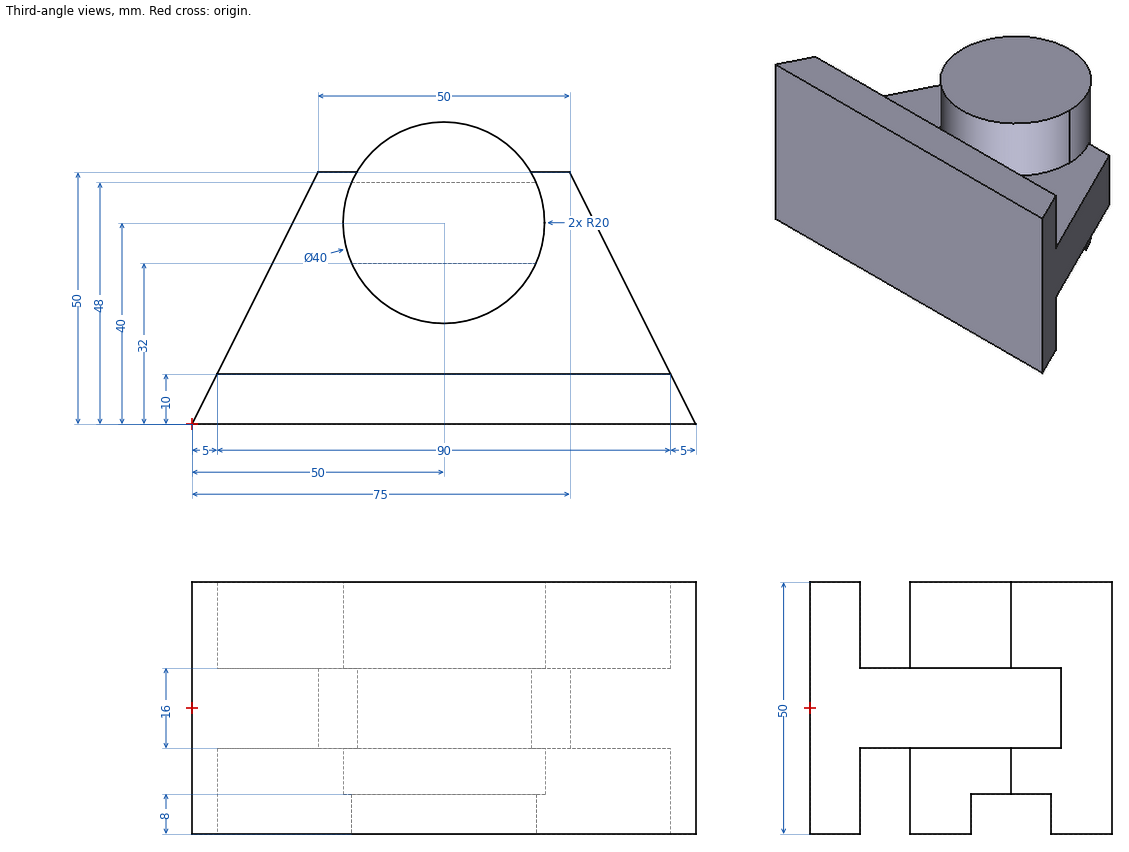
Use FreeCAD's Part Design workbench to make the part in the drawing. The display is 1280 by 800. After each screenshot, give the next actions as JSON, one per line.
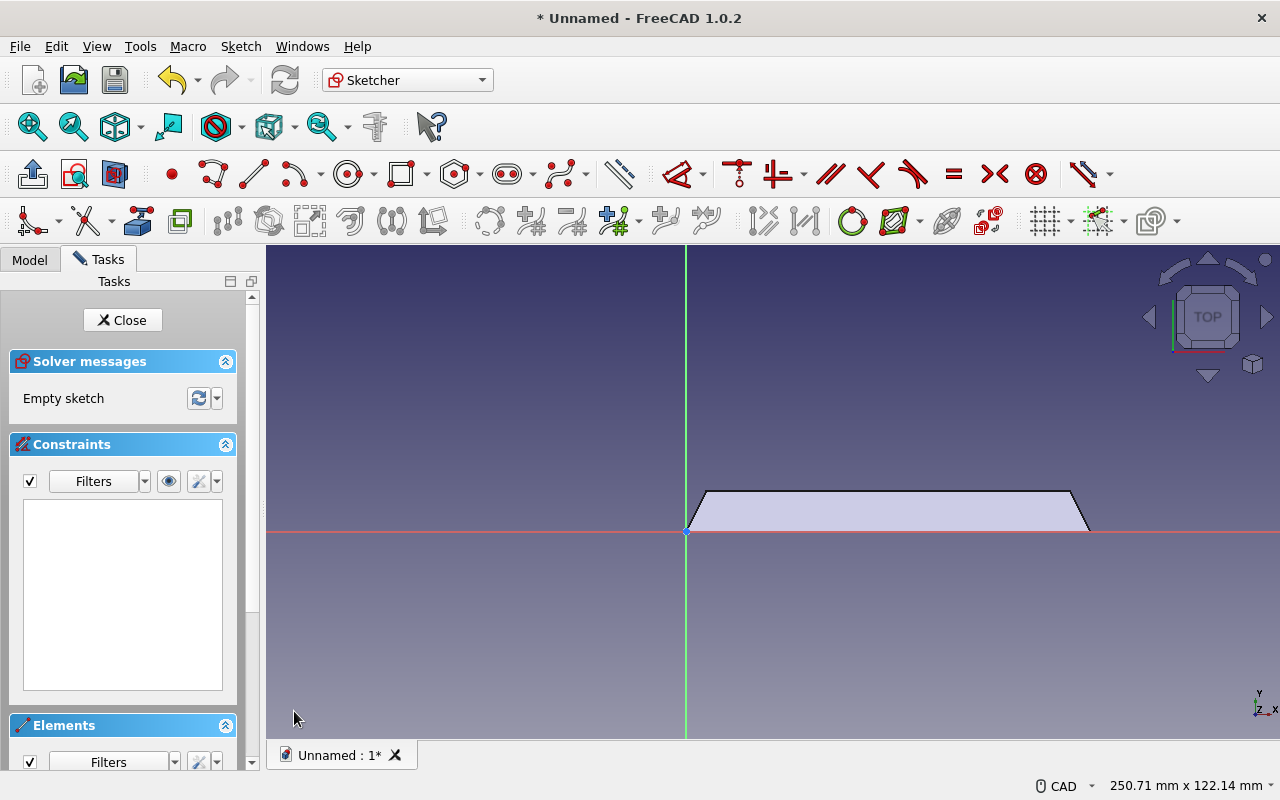
{"action": "scroll", "coordinate": [1115, 306], "scroll_direction": "up", "scroll_amount": 2}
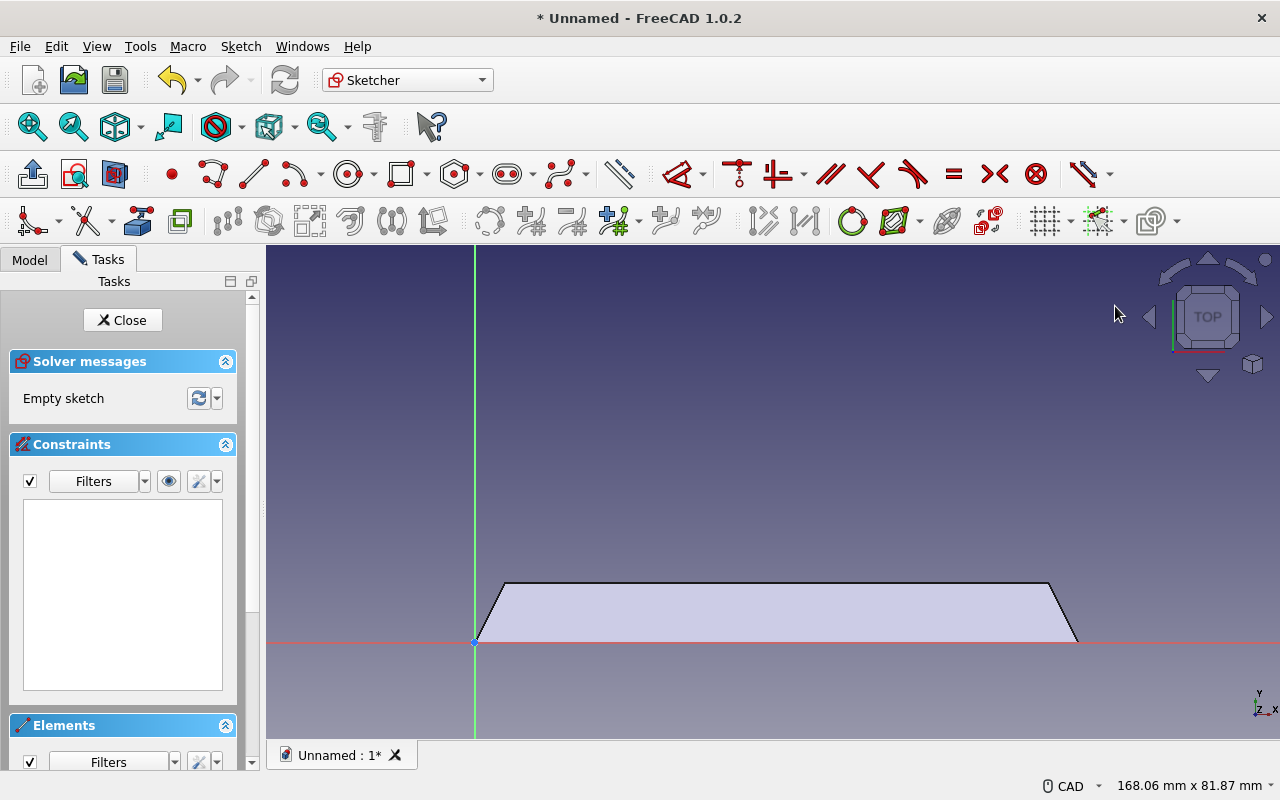
{"action": "left_click", "coordinate": [213, 174]}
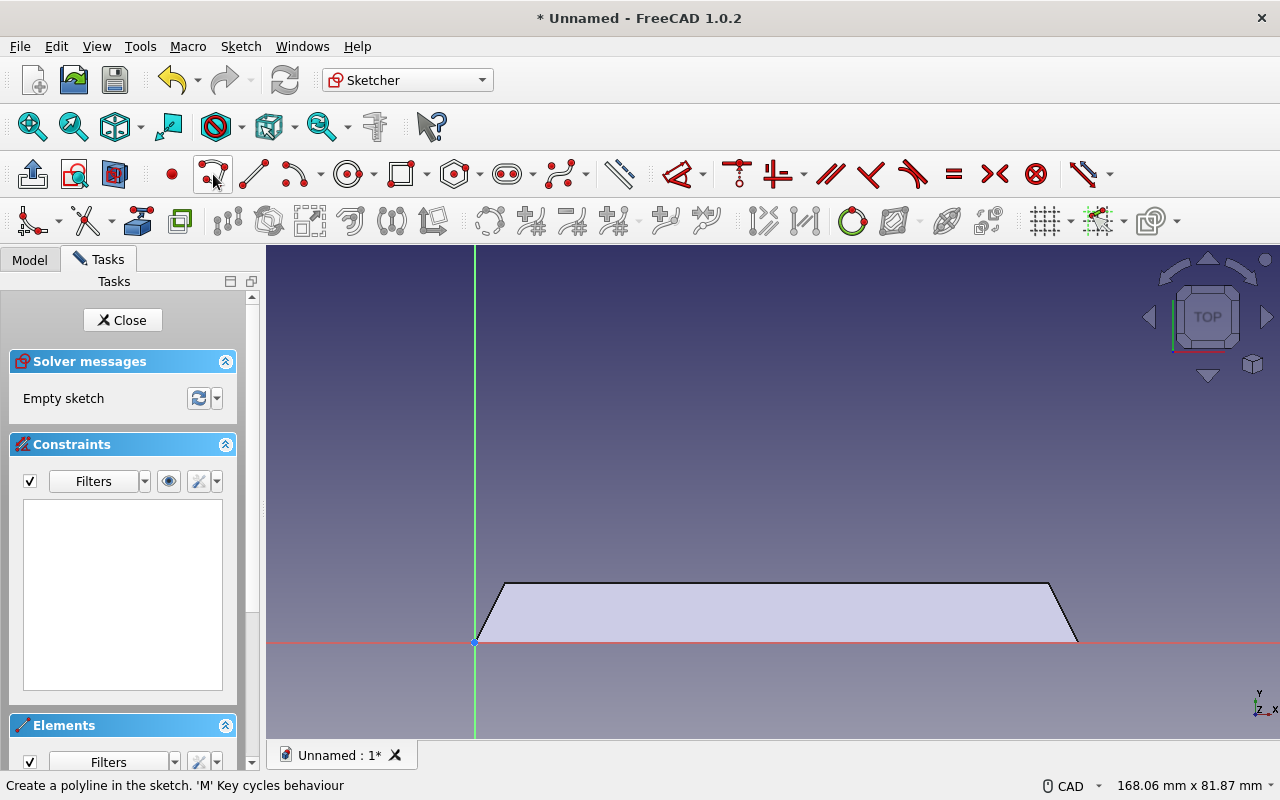
{"action": "left_click", "coordinate": [505, 583]}
{"action": "left_click", "coordinate": [1048, 583]}
{"action": "left_click", "coordinate": [927, 341]}
{"action": "left_click", "coordinate": [626, 341]}
{"action": "left_click", "coordinate": [505, 584]}
{"action": "key", "text": "Escape"}
{"action": "key", "text": "Escape"}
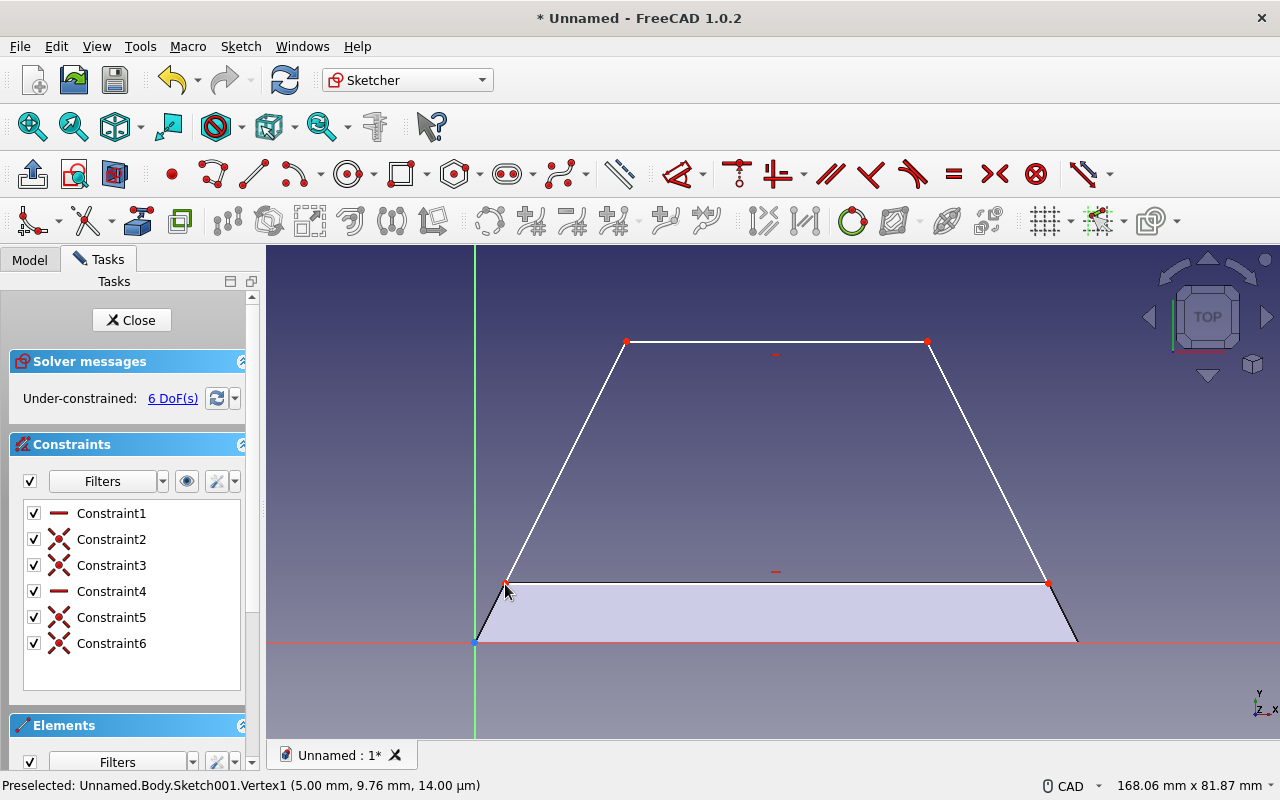
{"action": "left_click", "coordinate": [676, 174]}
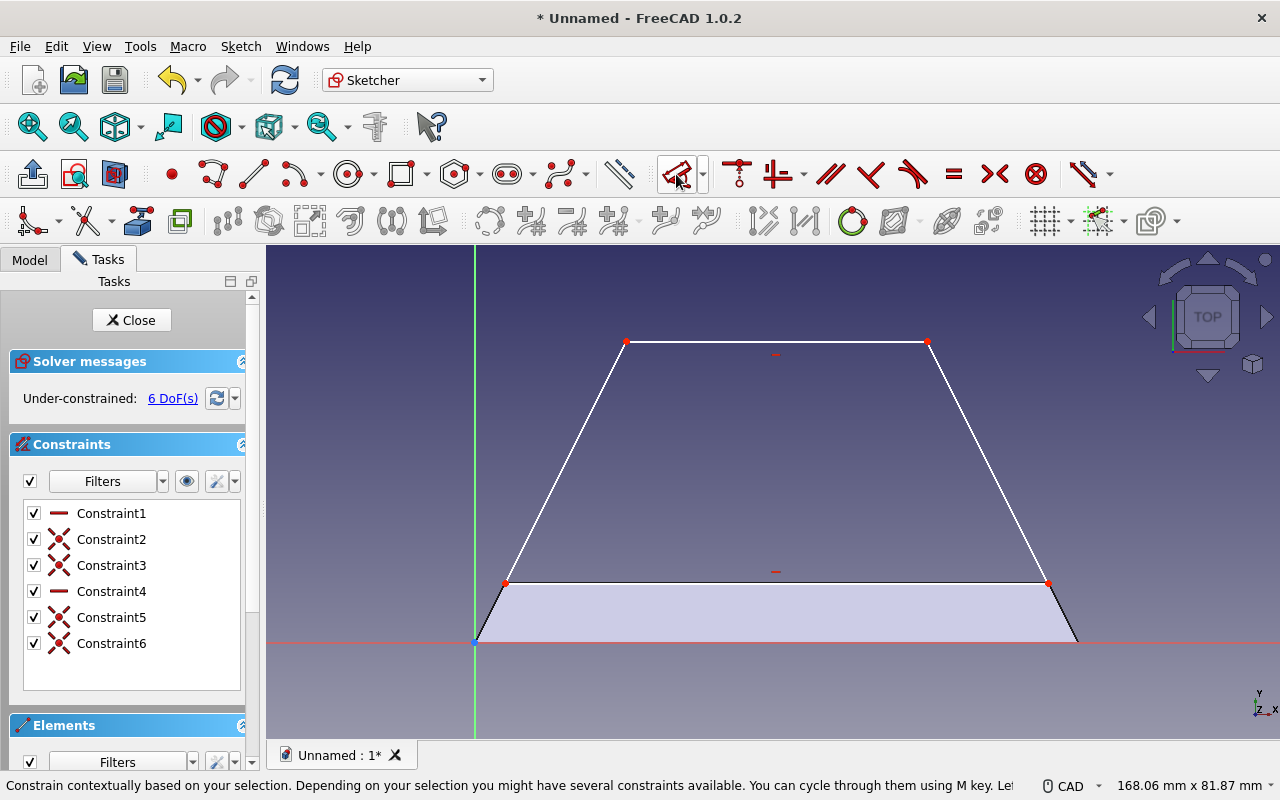
{"action": "left_click", "coordinate": [668, 584]}
{"action": "left_click", "coordinate": [776, 618]}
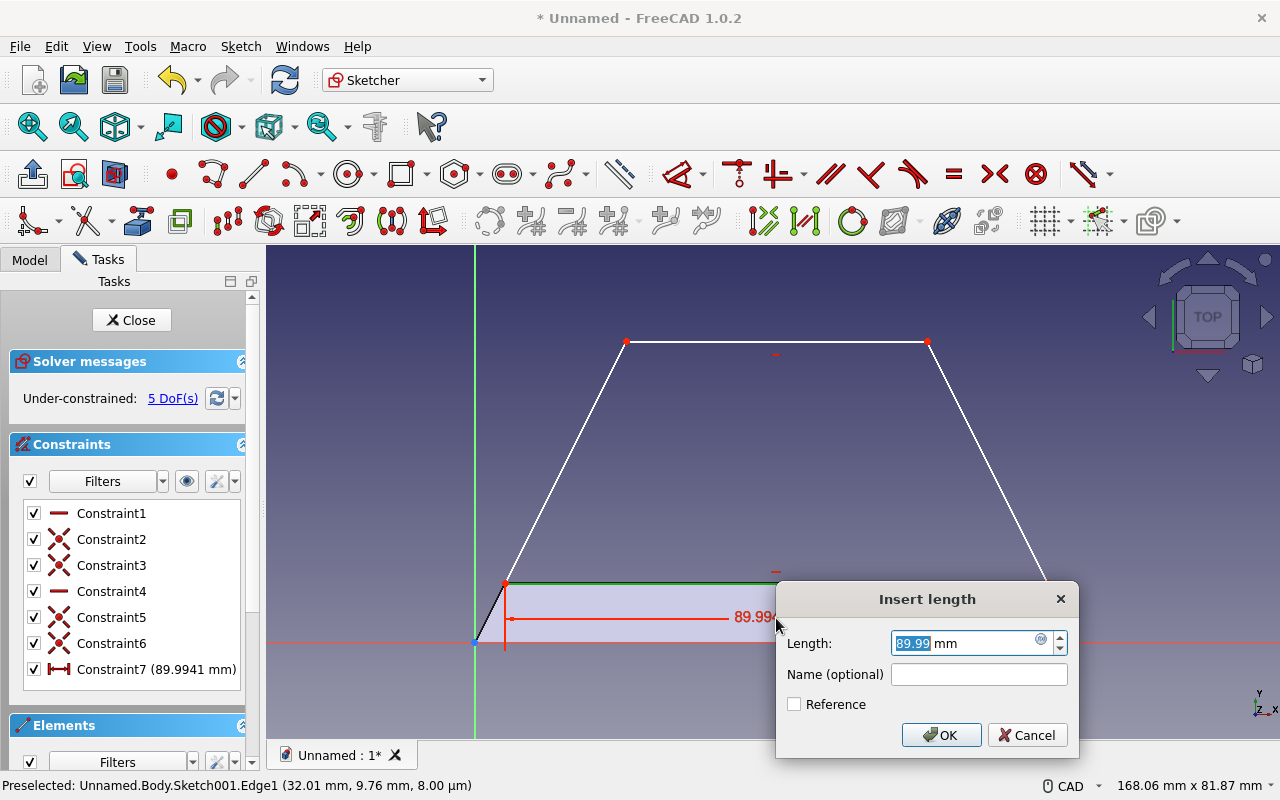
{"action": "type", "text": "90"}
{"action": "key", "text": "Return"}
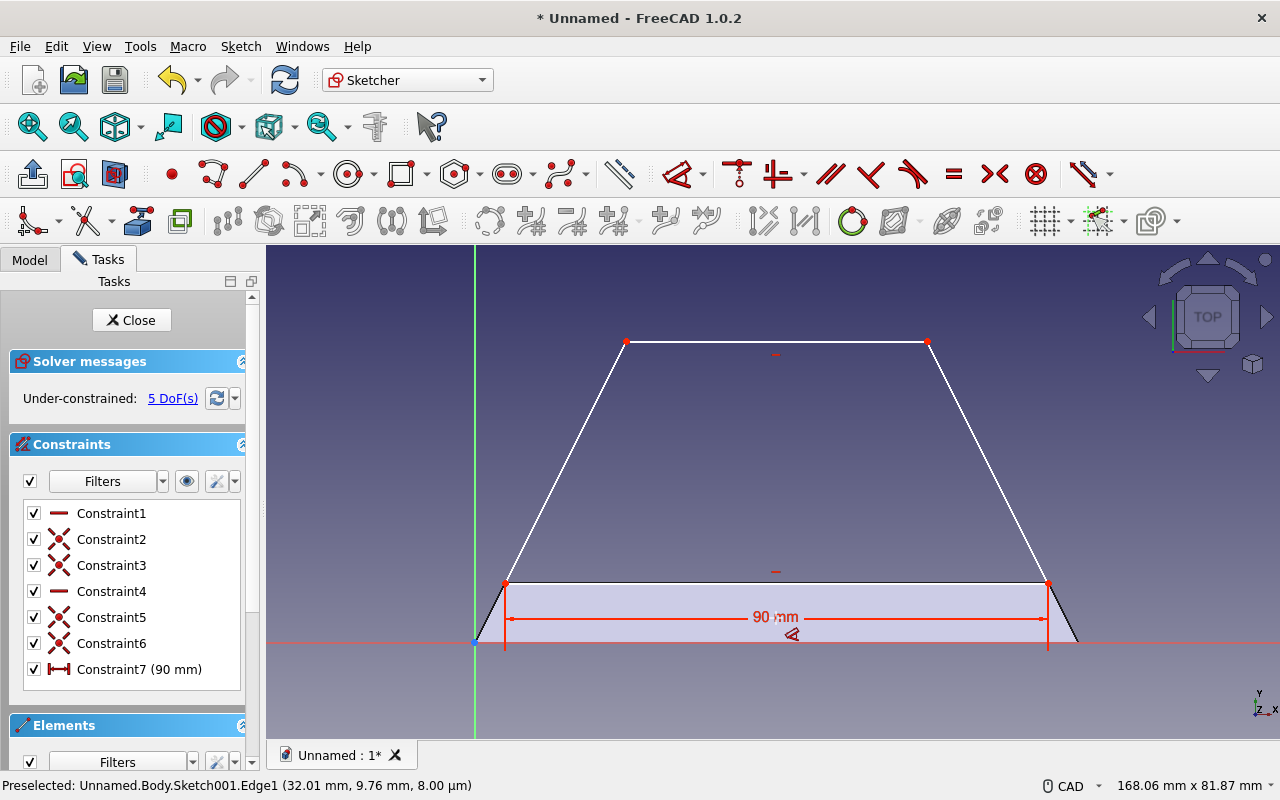
{"action": "left_click", "coordinate": [837, 342]}
{"action": "left_click", "coordinate": [777, 308]}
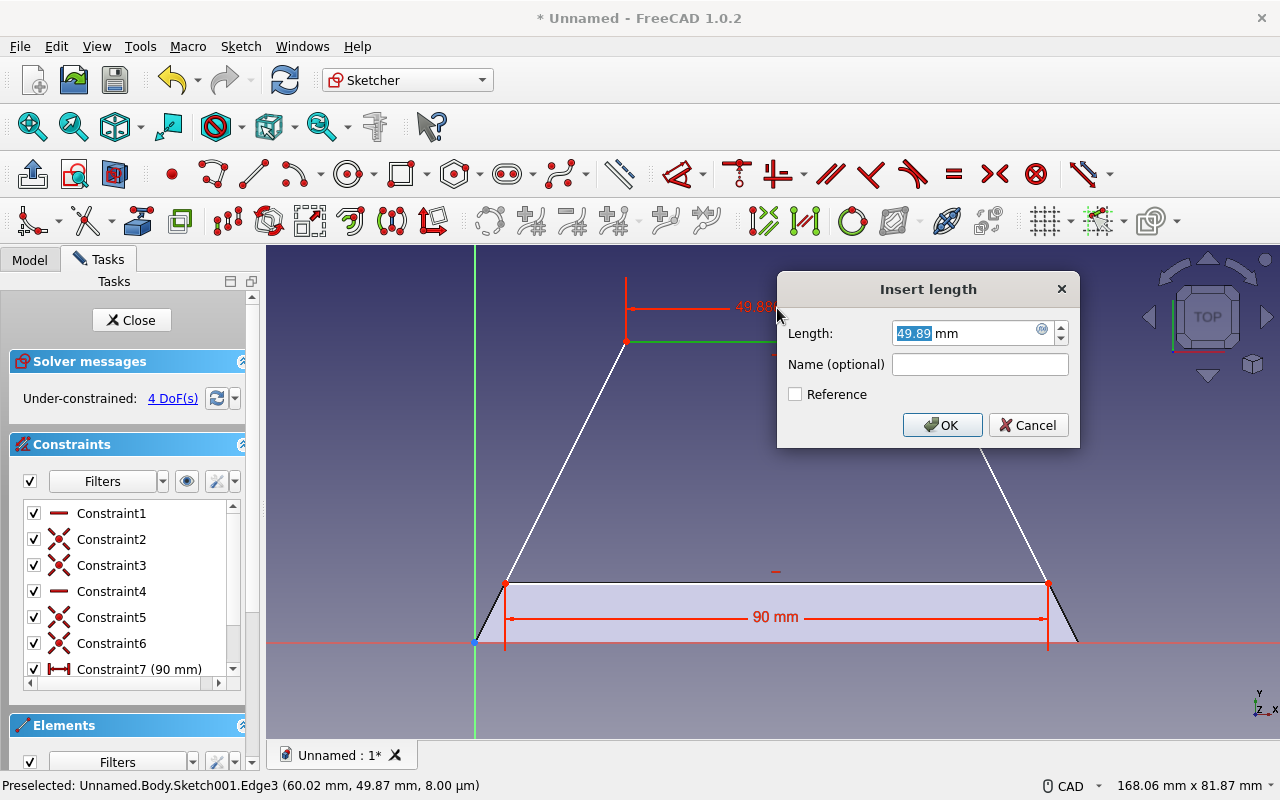
{"action": "type", "text": "50"}
{"action": "key", "text": "Return"}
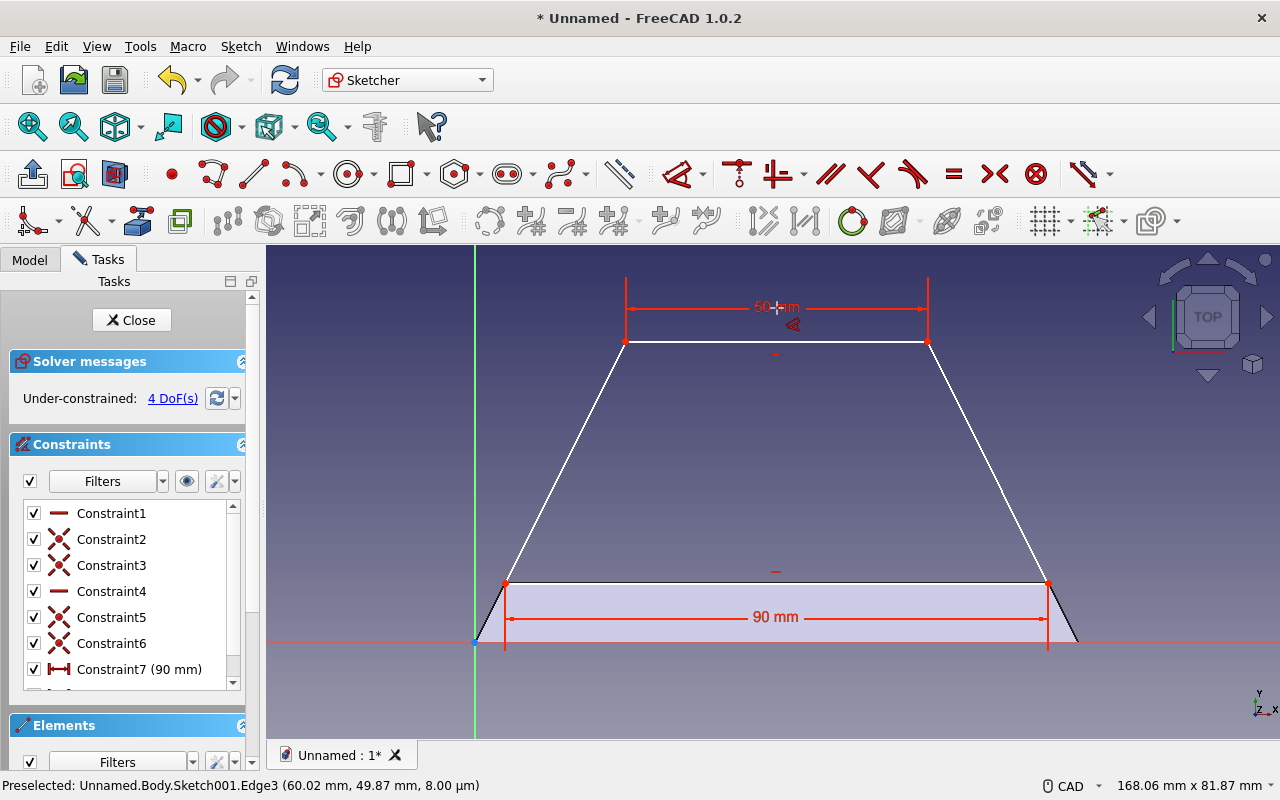
{"action": "scroll", "coordinate": [505, 584], "scroll_direction": "up", "scroll_amount": 2}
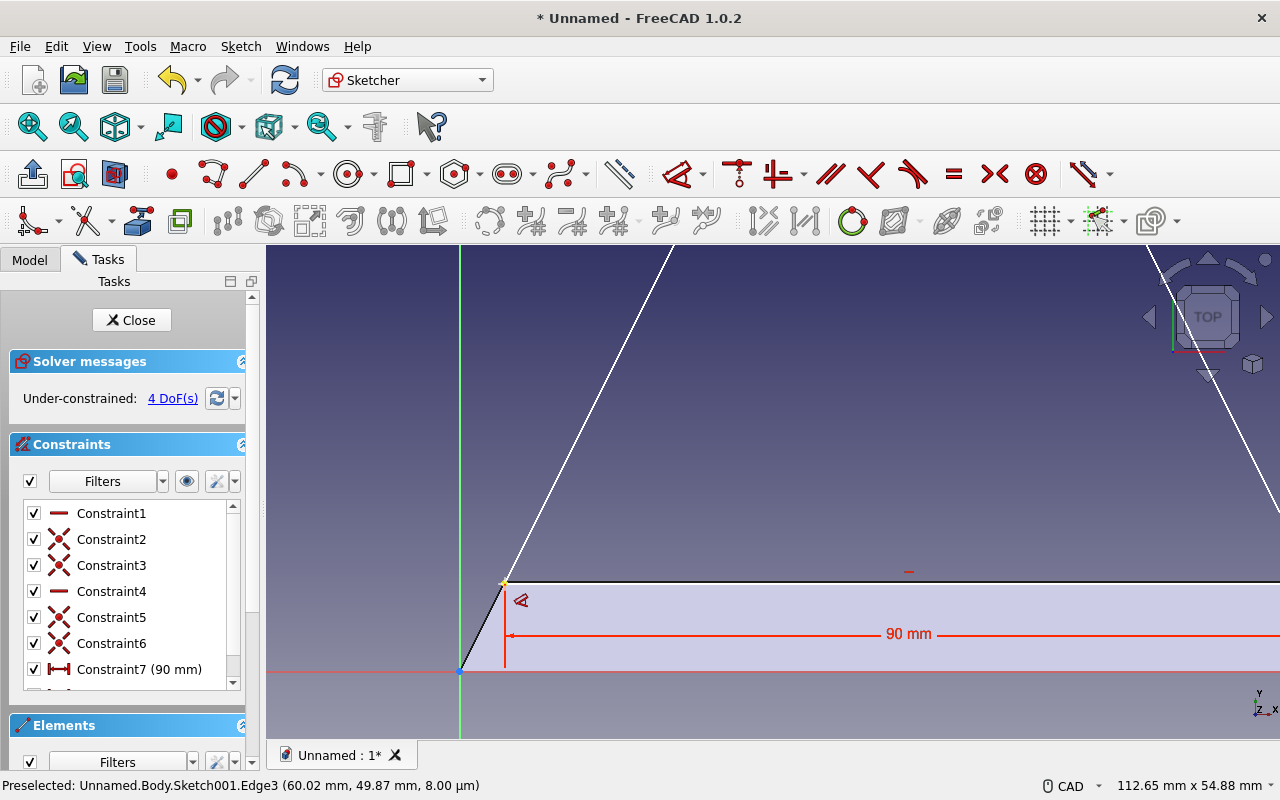
{"action": "left_click", "coordinate": [505, 584]}
{"action": "left_click", "coordinate": [482, 706]}